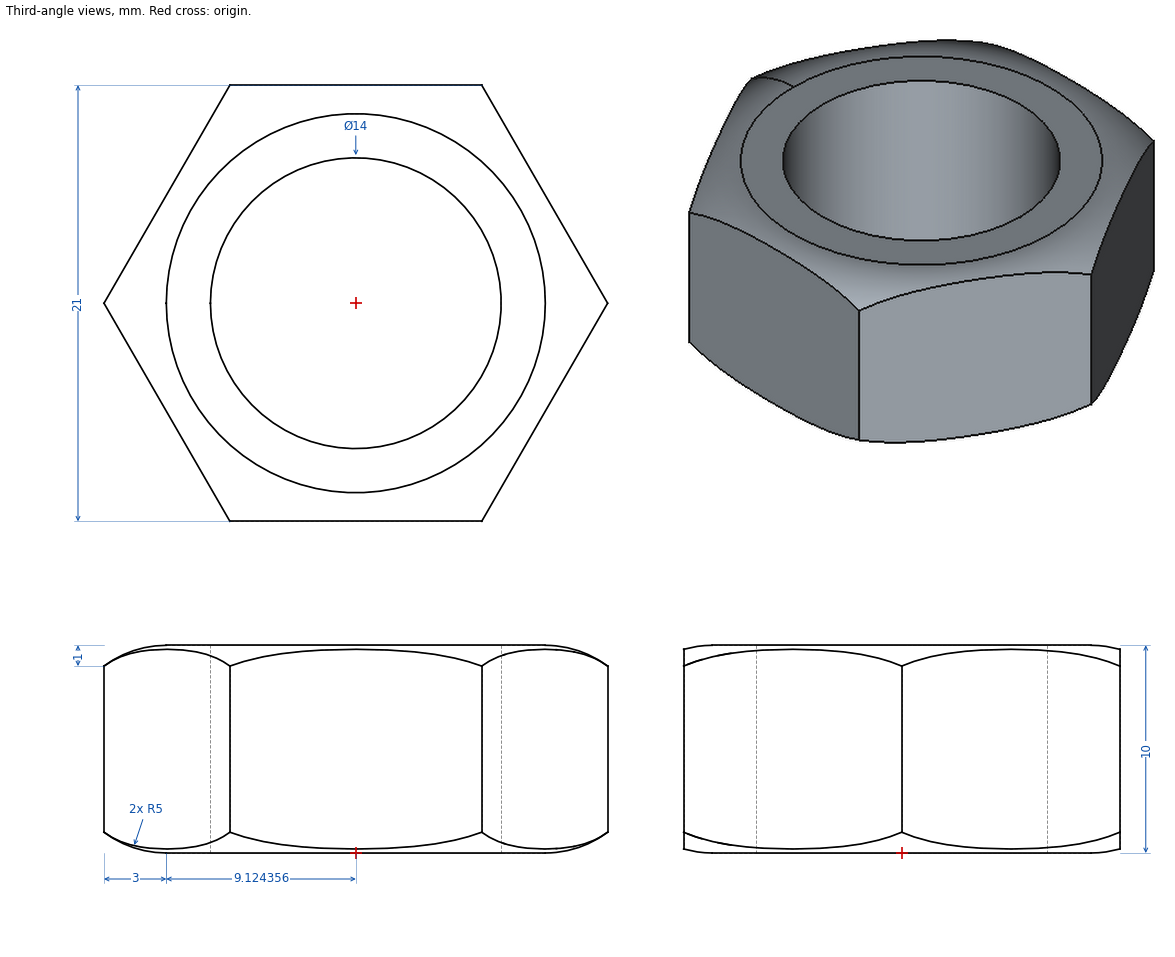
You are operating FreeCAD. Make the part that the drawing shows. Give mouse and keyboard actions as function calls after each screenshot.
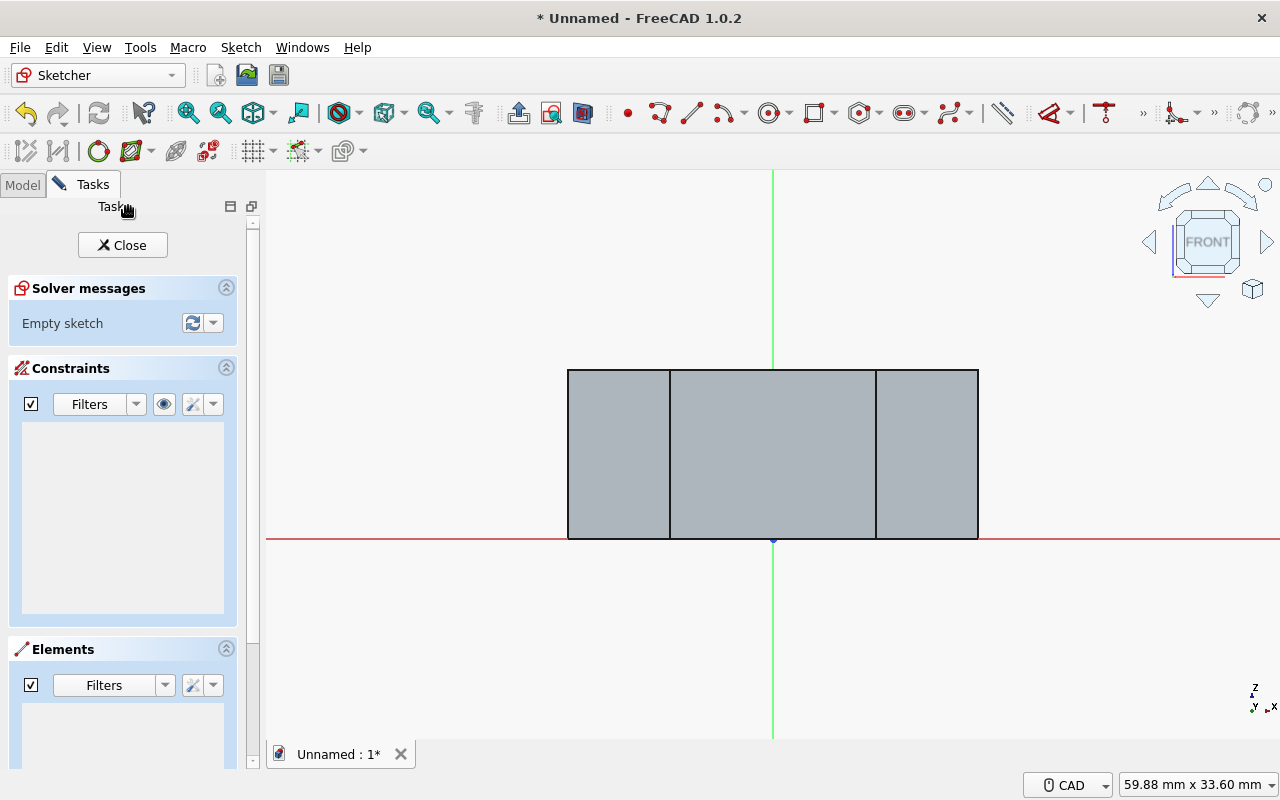
click(584, 114)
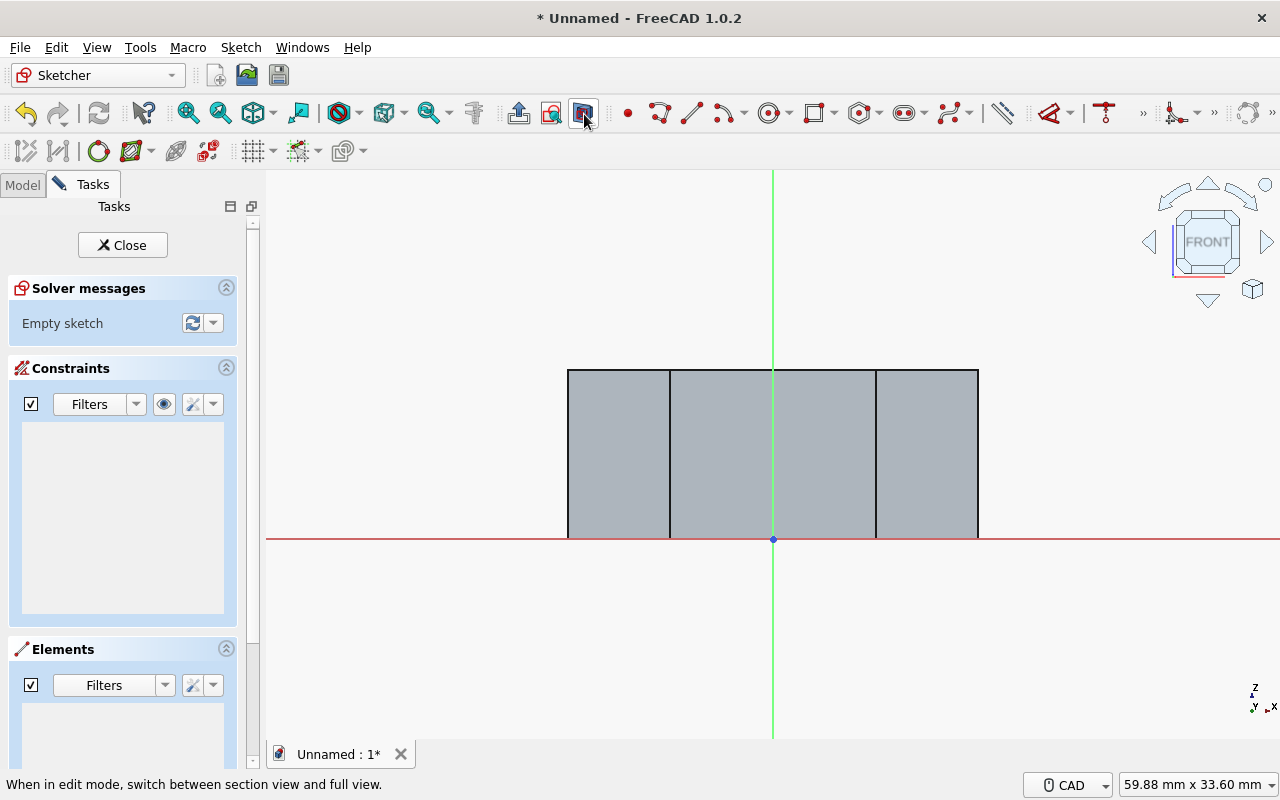
scroll(642, 455, up, 4)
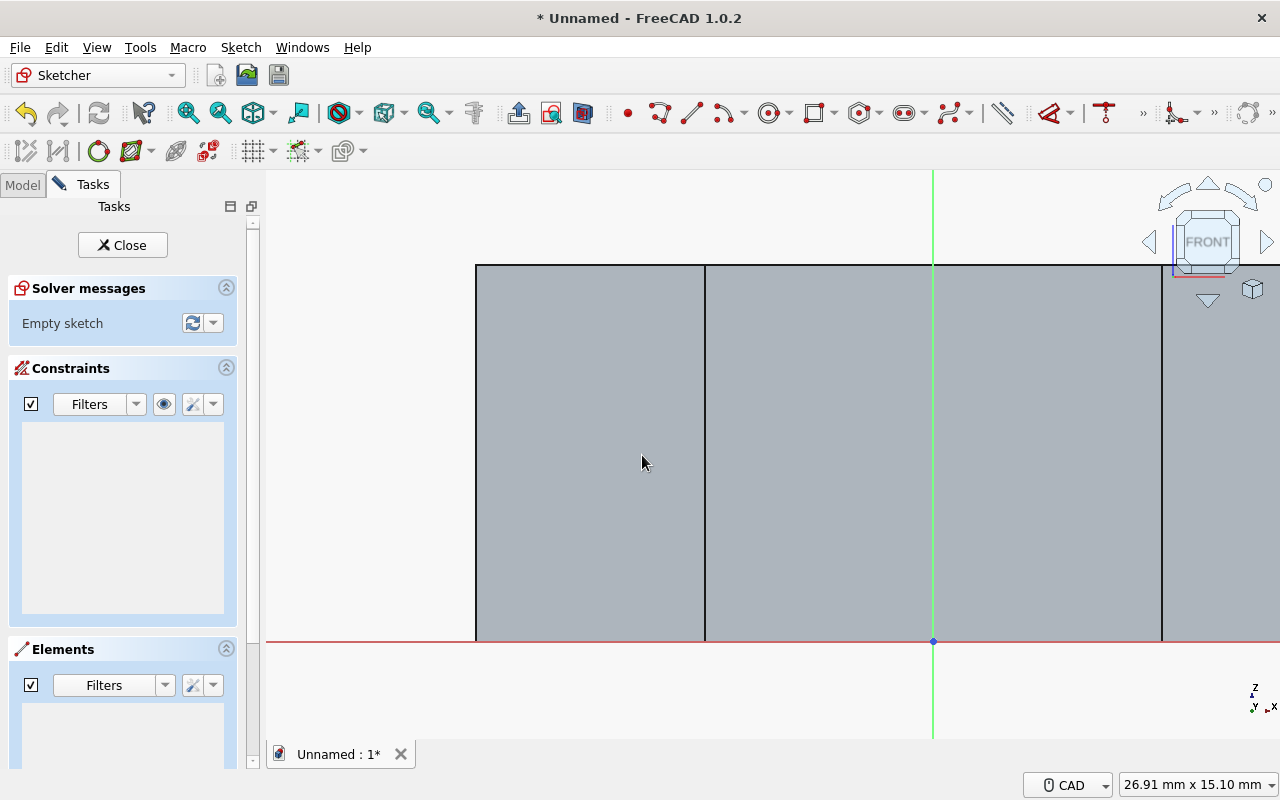
click(660, 114)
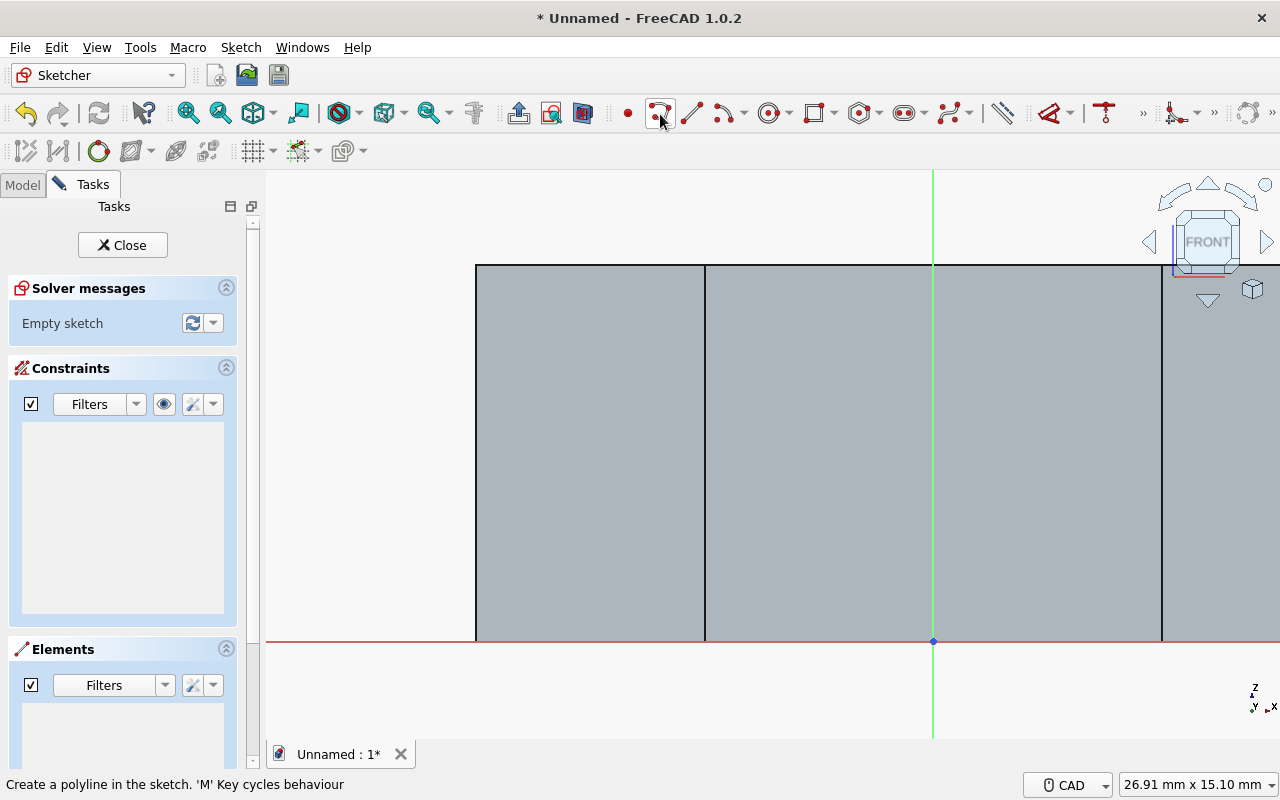
click(589, 642)
click(476, 633)
click(476, 604)
right_click(476, 604)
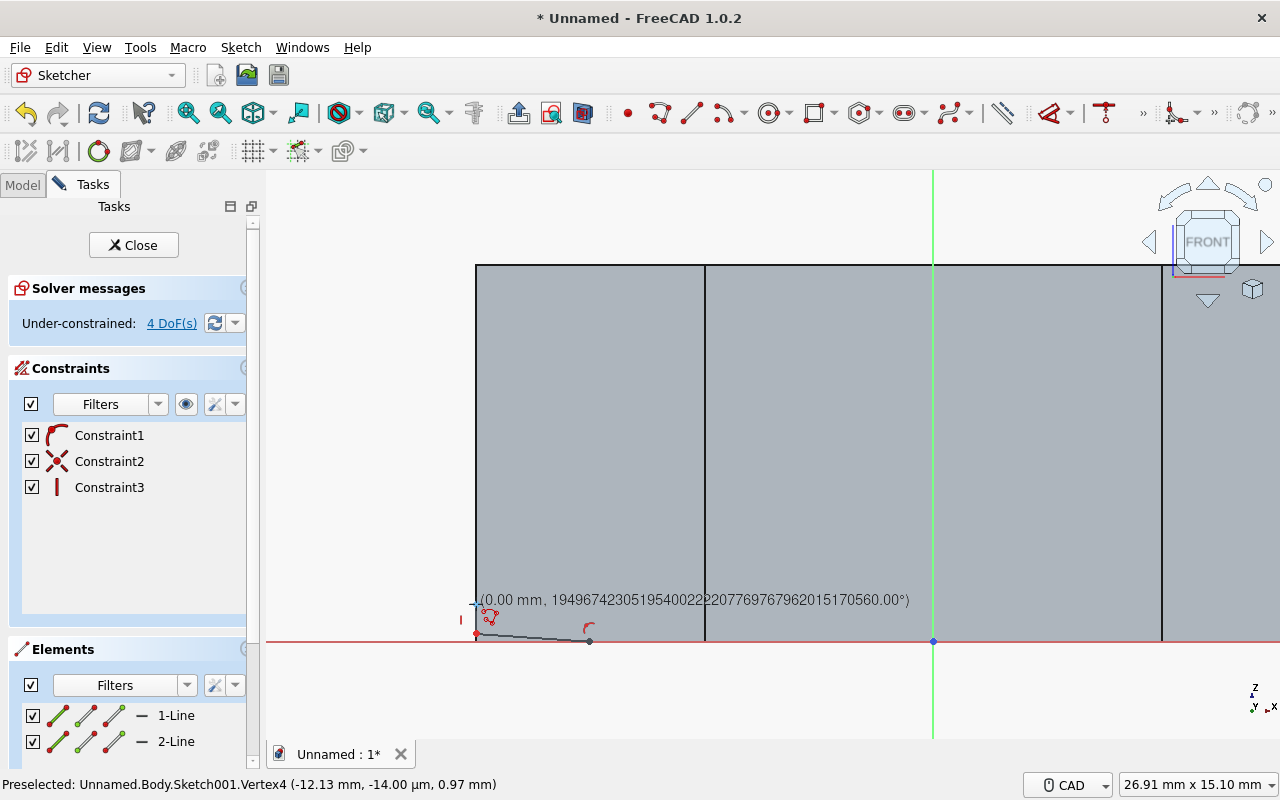
key(g)
key(3)
key(a)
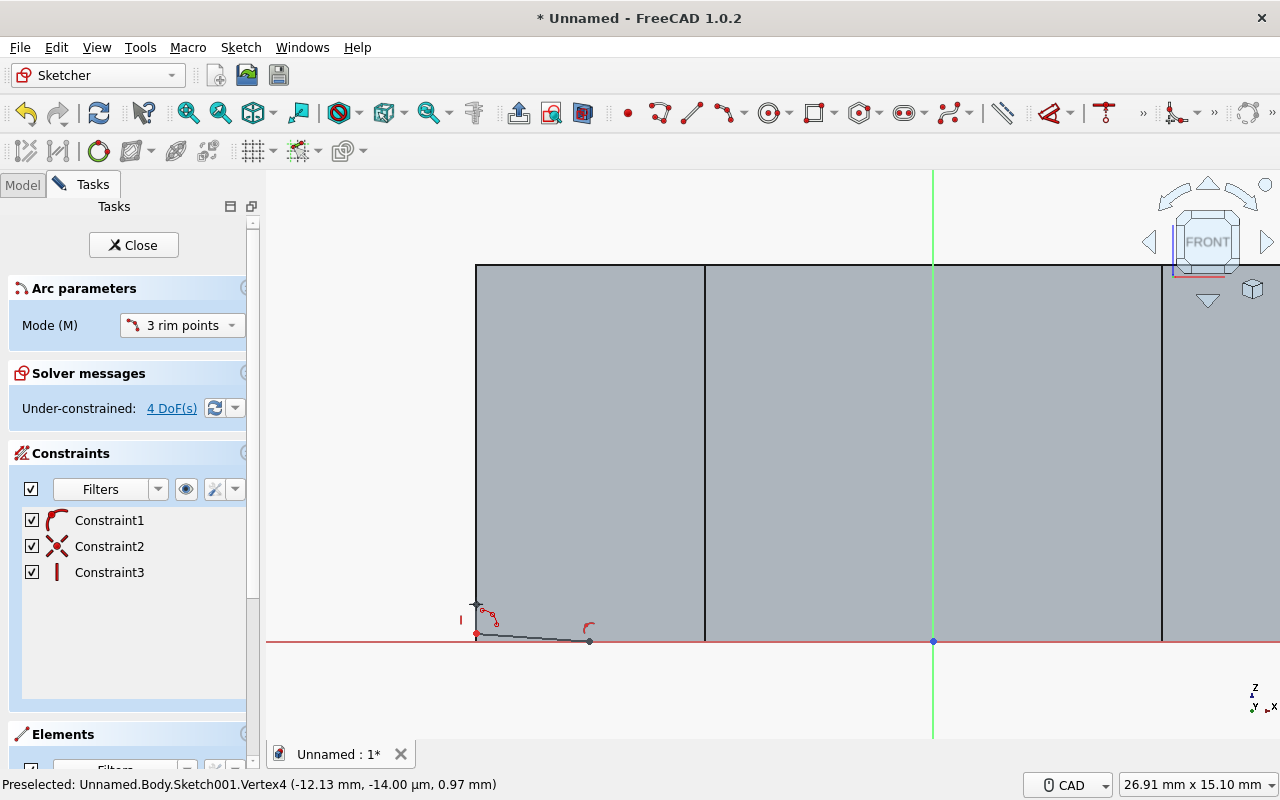
click(476, 605)
click(589, 642)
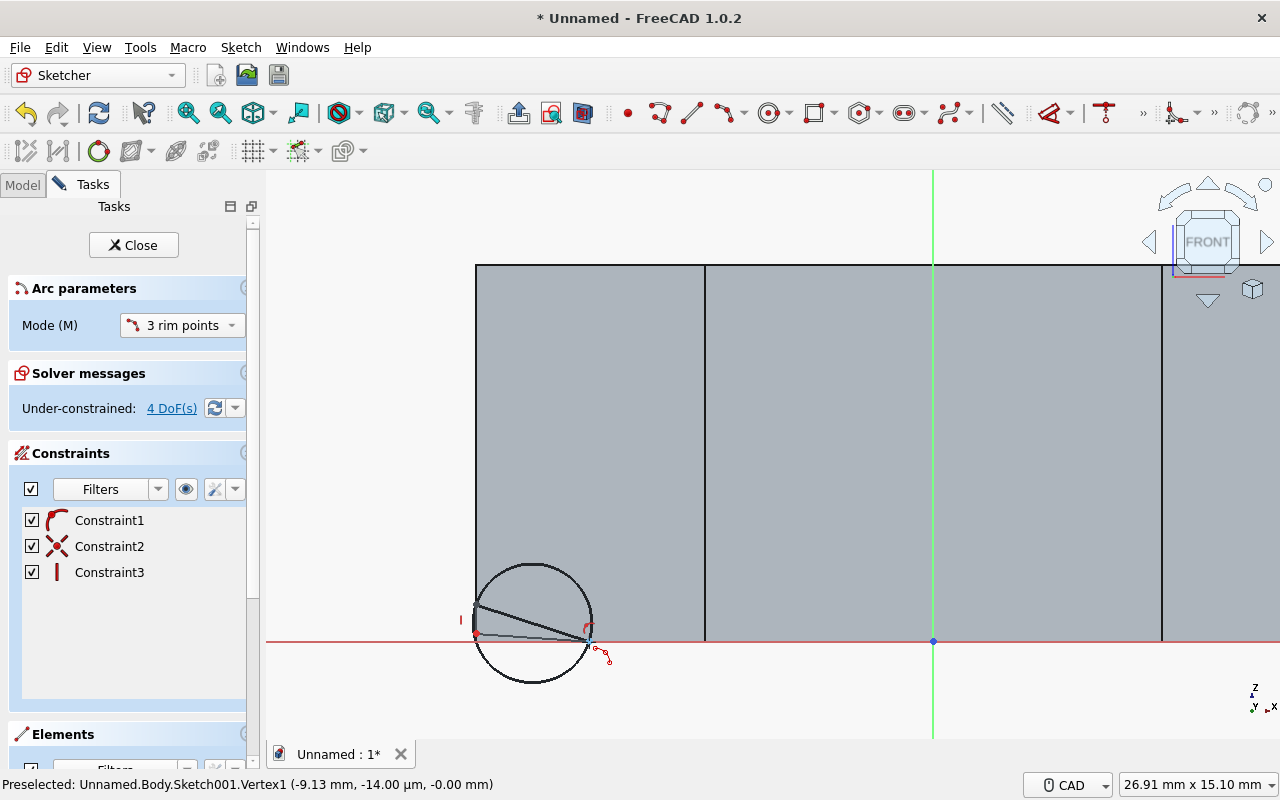
scroll(530, 632, up, 3)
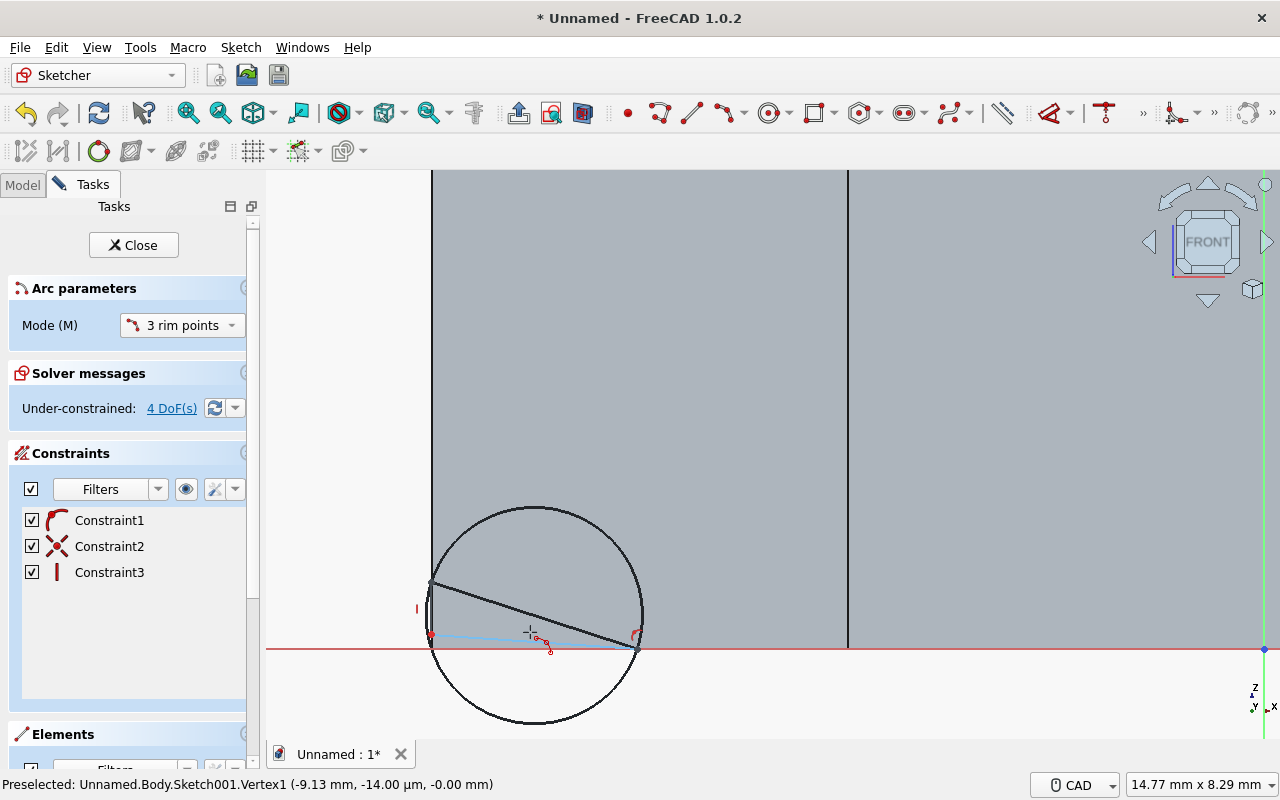
click(529, 631)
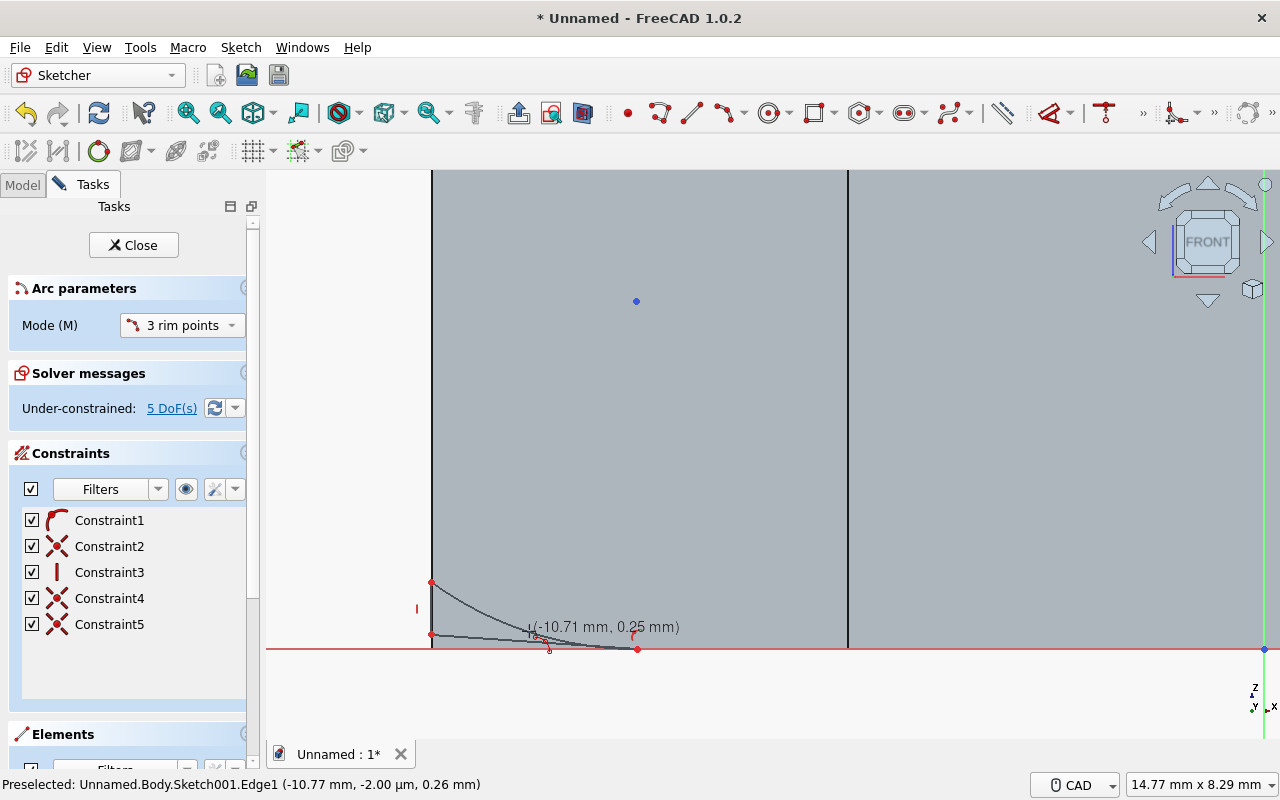
key(g)
key(m)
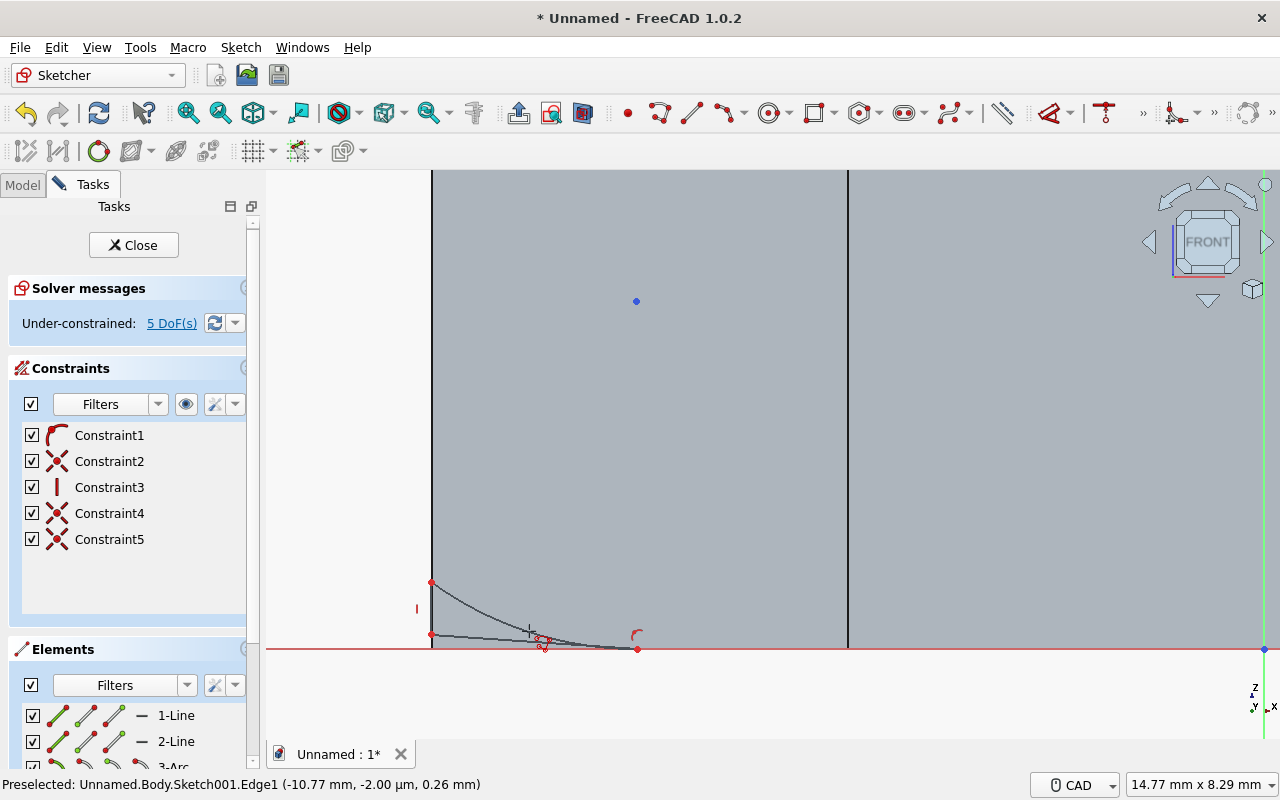
scroll(530, 636, down, 3)